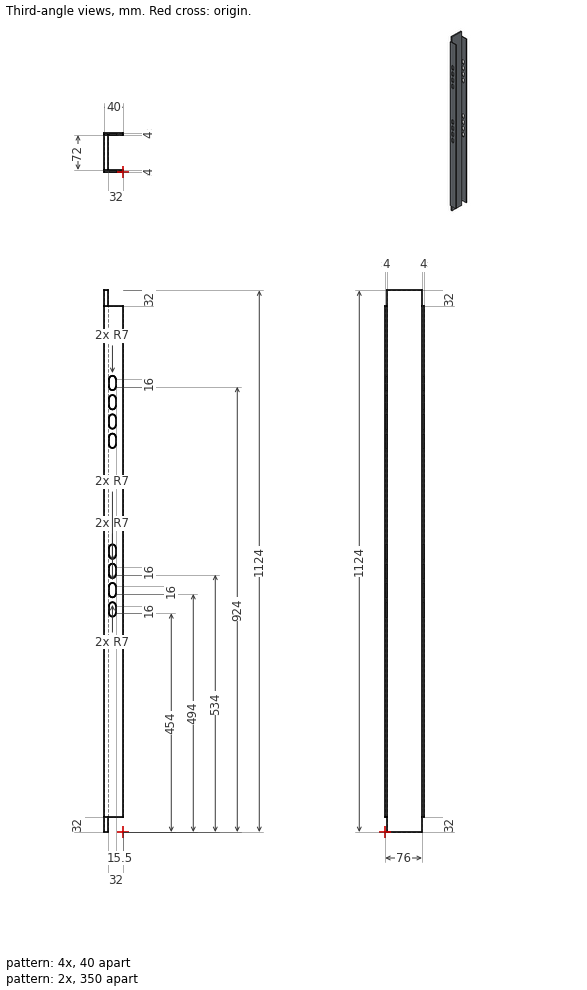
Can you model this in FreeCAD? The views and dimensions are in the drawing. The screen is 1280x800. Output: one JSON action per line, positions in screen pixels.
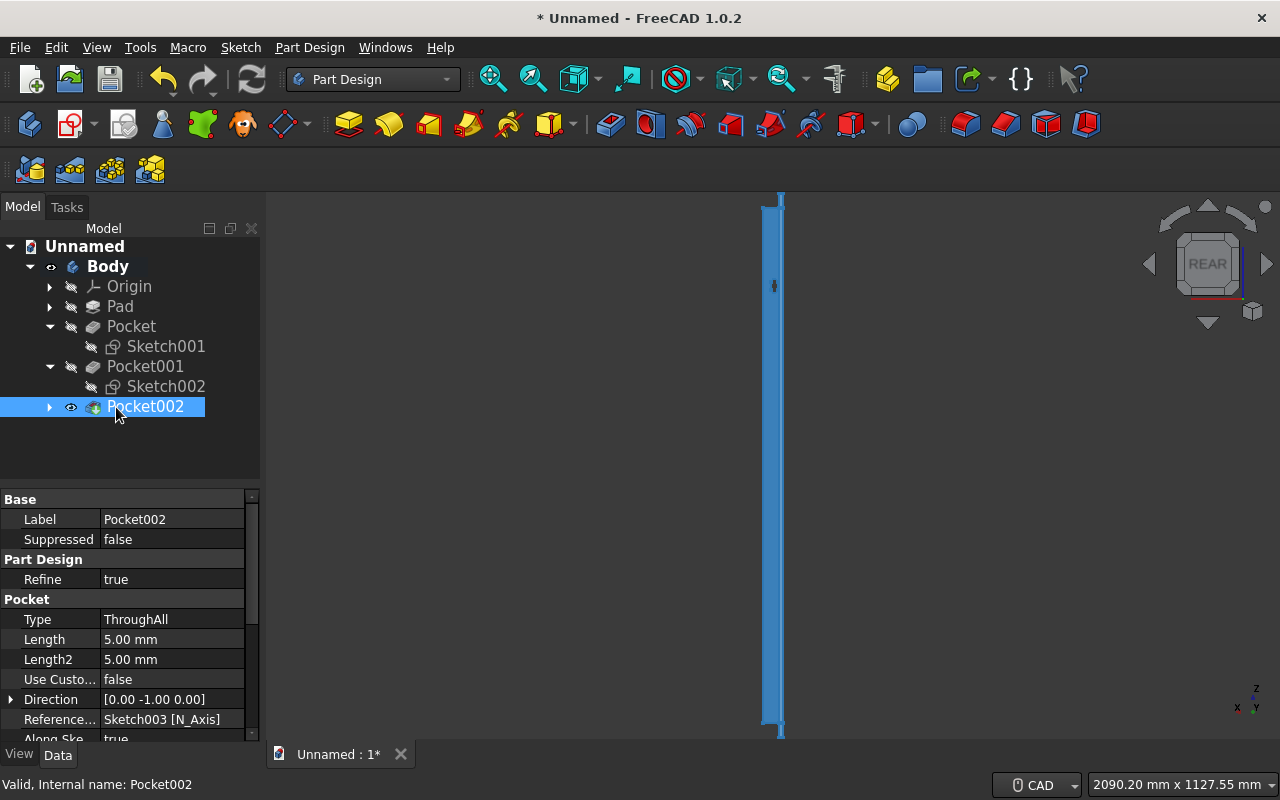
{"action": "left_click", "coordinate": [70, 170]}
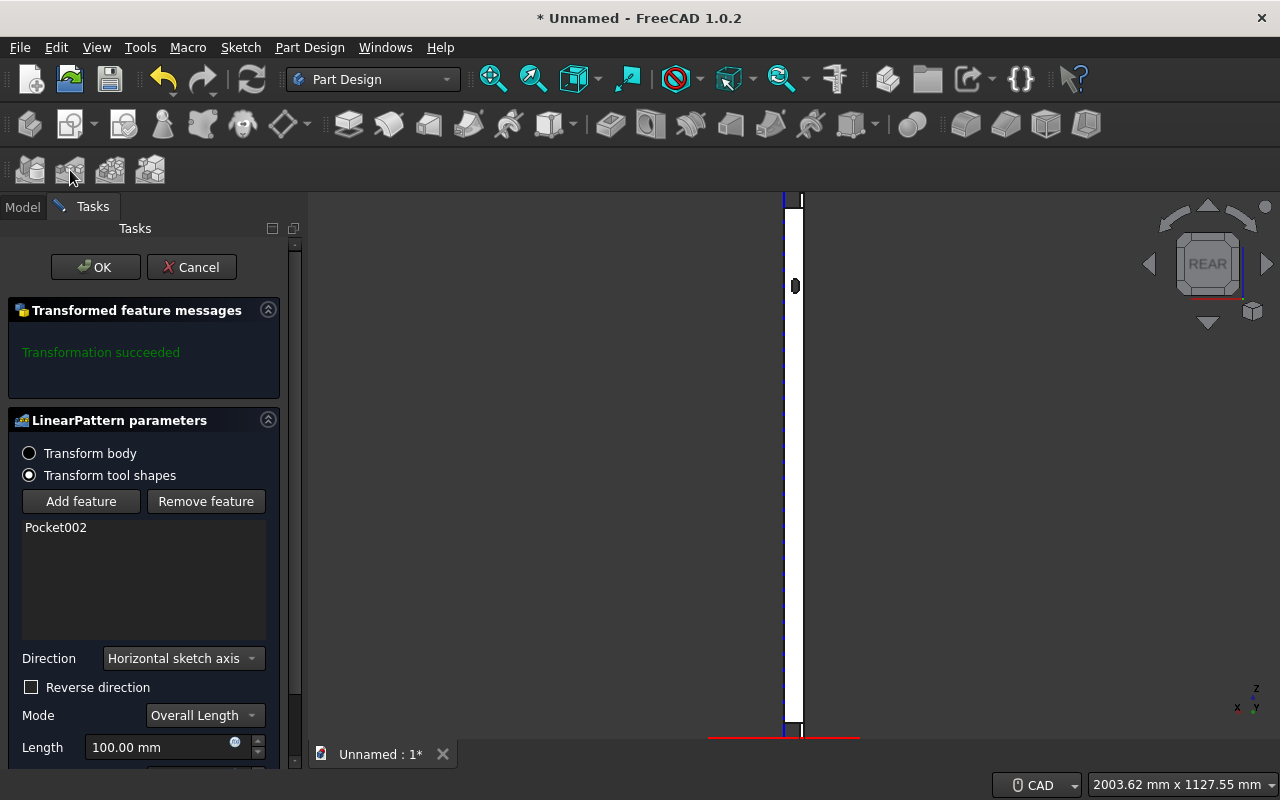
{"action": "left_click", "coordinate": [184, 658]}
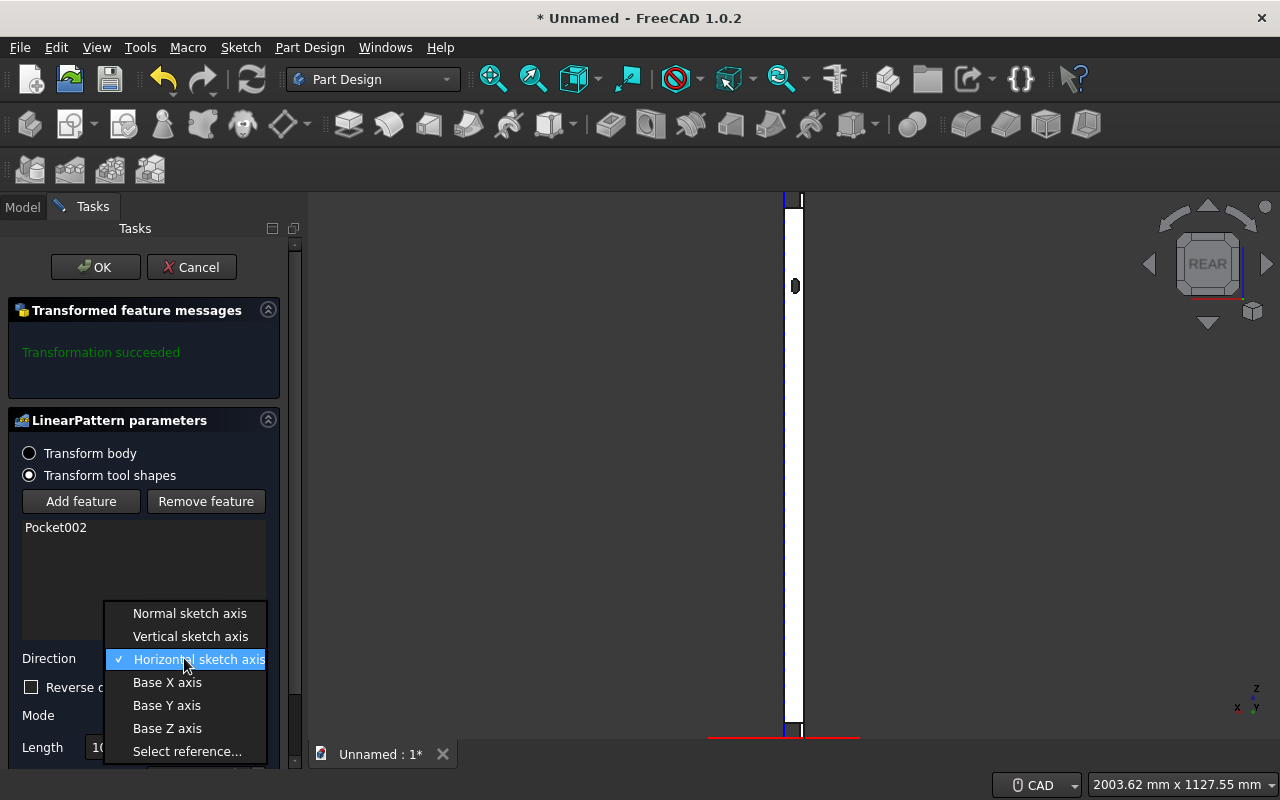
{"action": "left_click", "coordinate": [184, 728]}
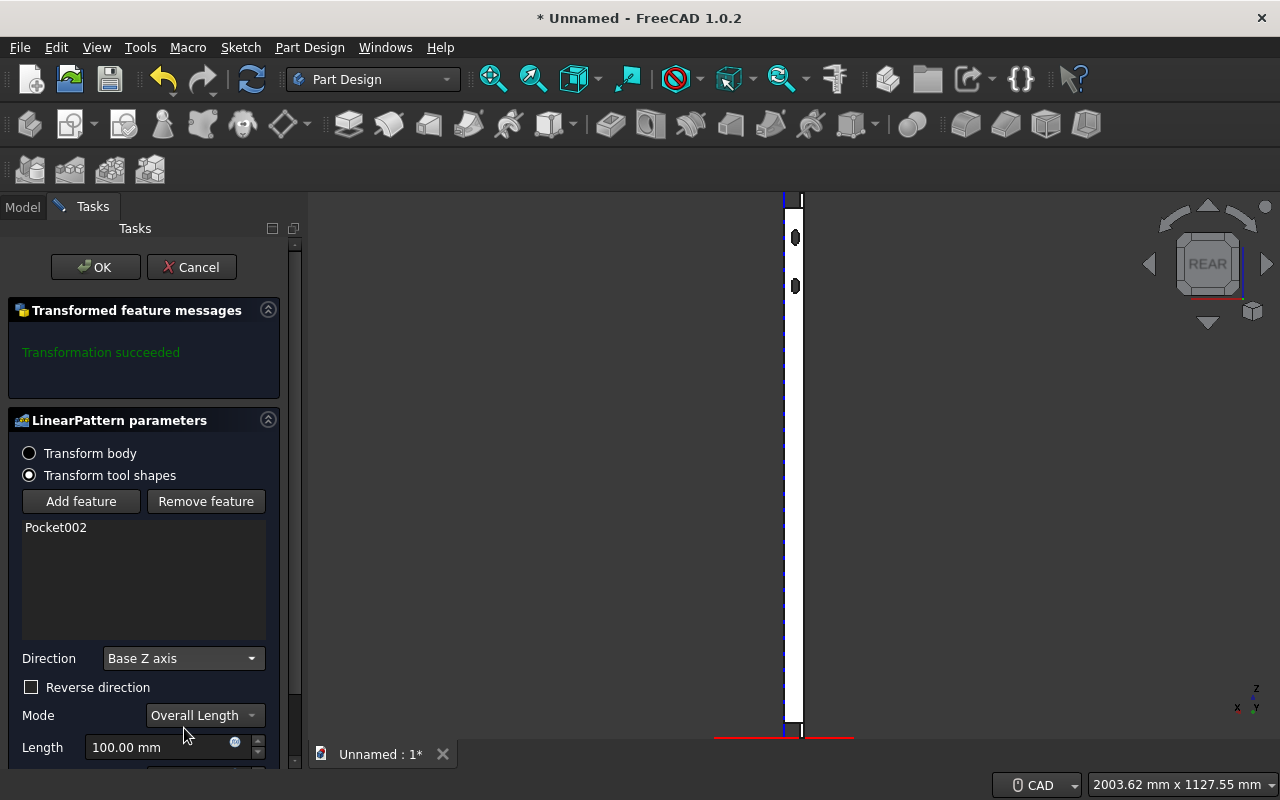
{"action": "left_click", "coordinate": [206, 716]}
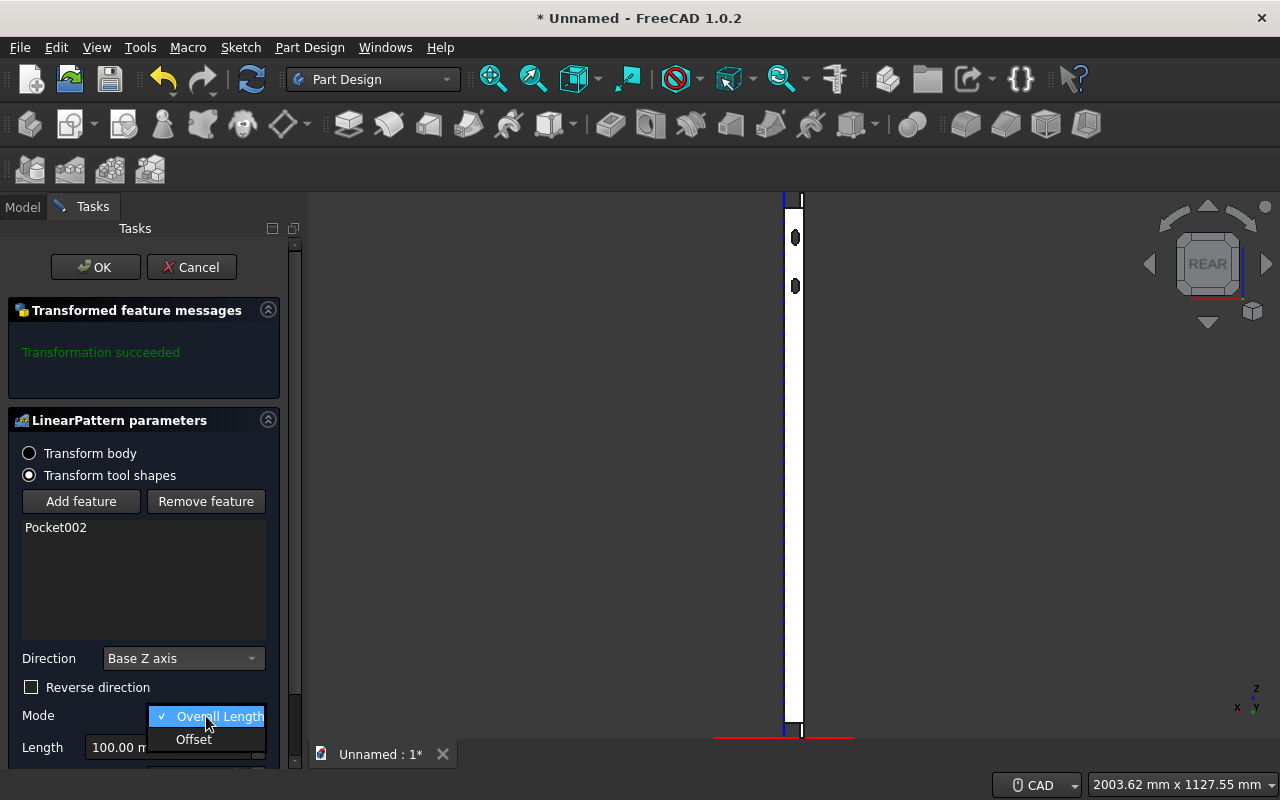
{"action": "left_click", "coordinate": [206, 740]}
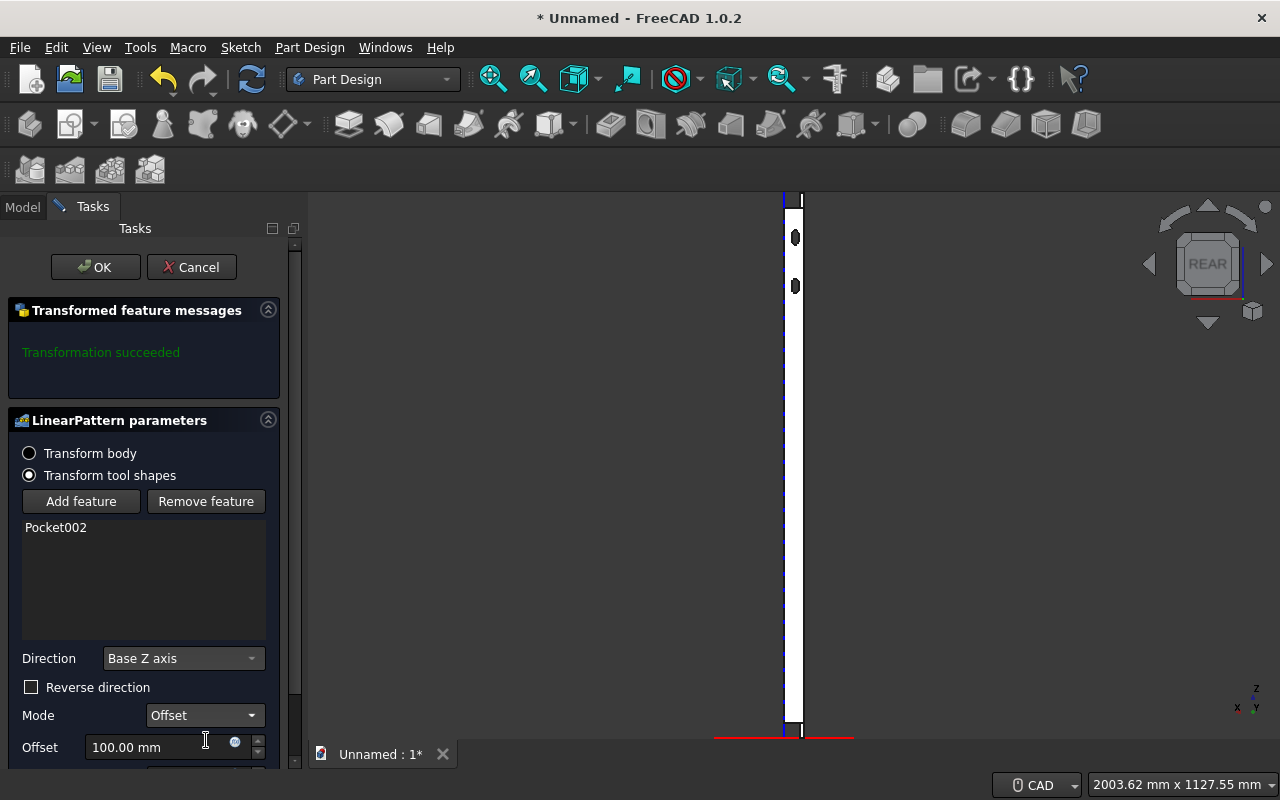
{"action": "triple_click", "coordinate": [168, 747]}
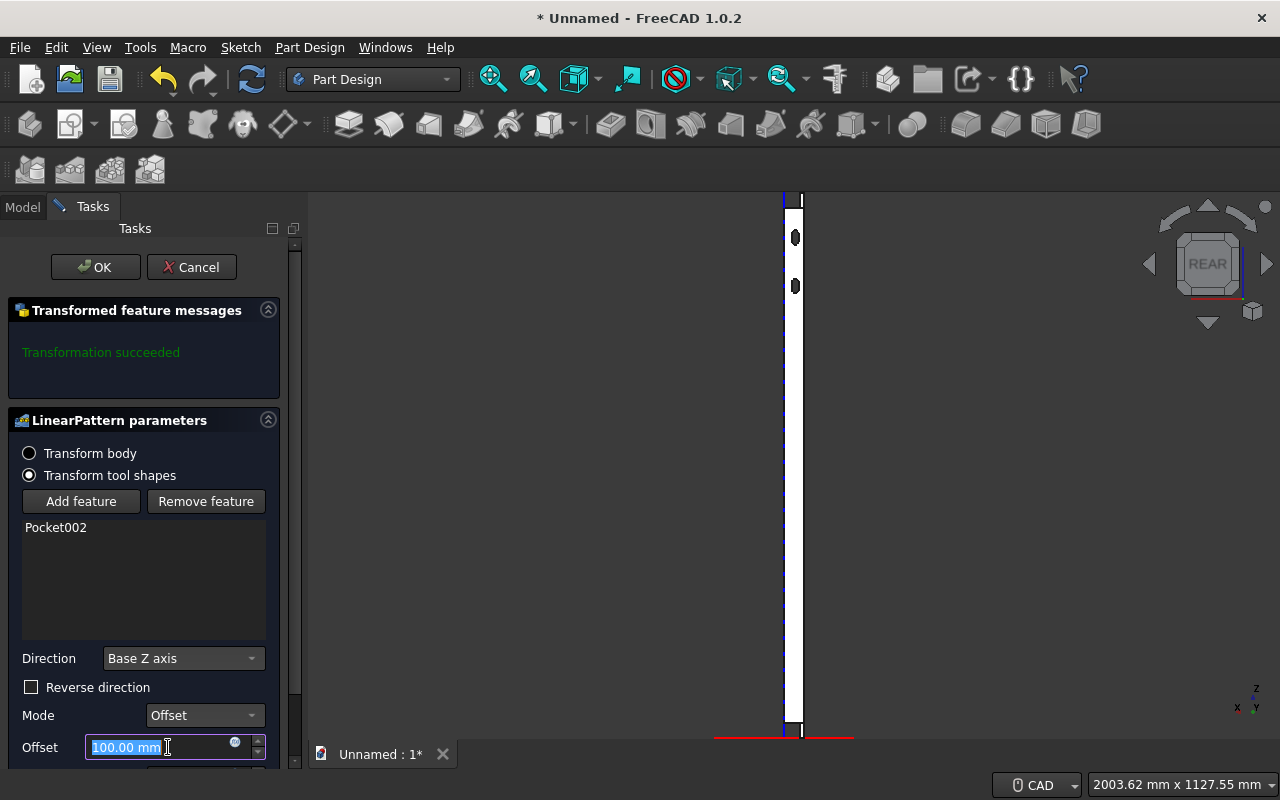
{"action": "type", "text": "40"}
{"action": "key", "text": "Tab"}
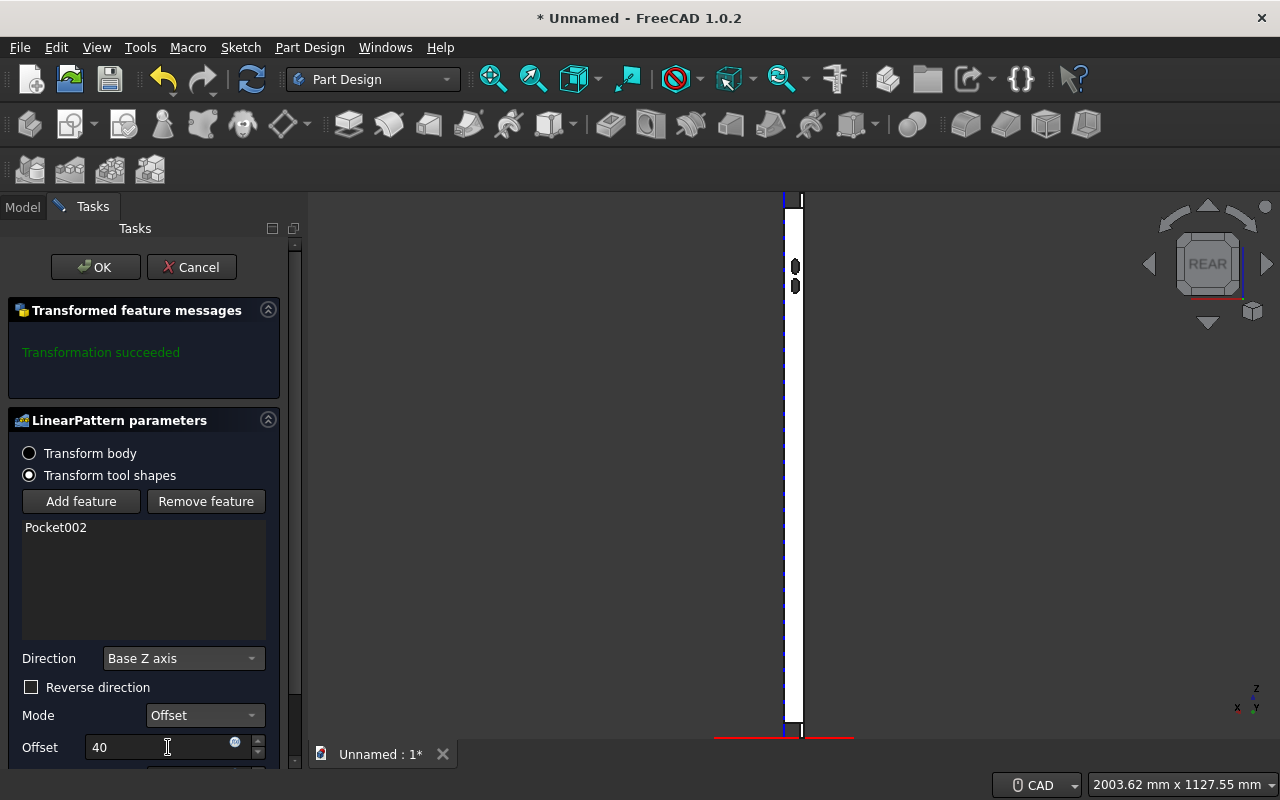
{"action": "scroll", "coordinate": [295, 503], "scroll_direction": "down", "scroll_amount": 2}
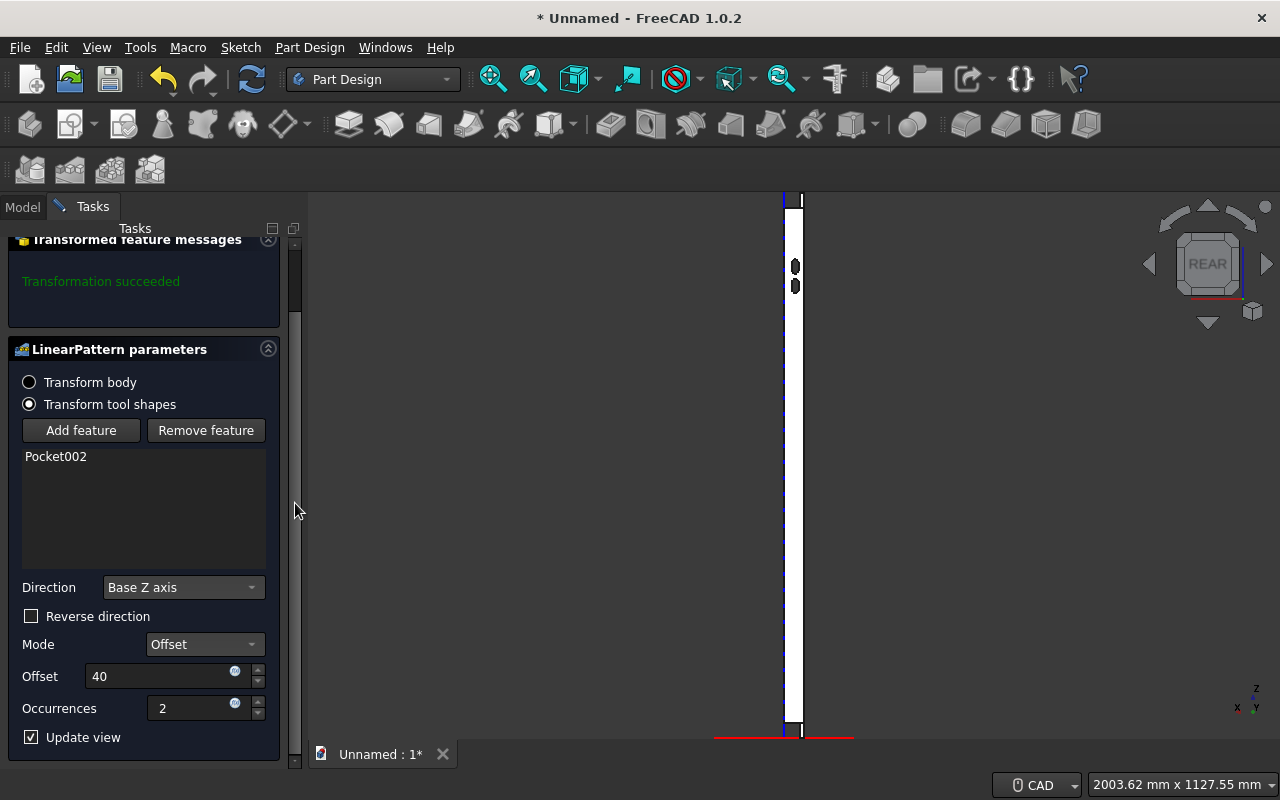
{"action": "triple_click", "coordinate": [198, 708]}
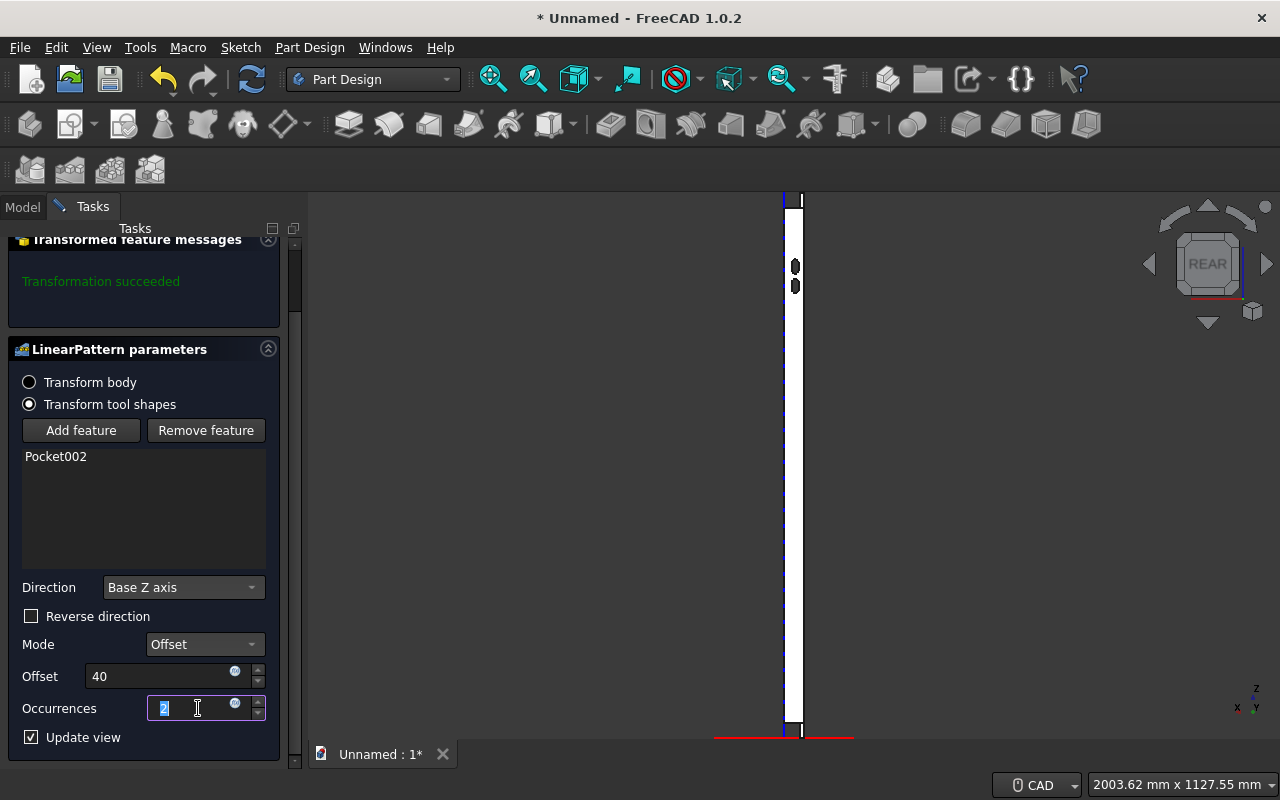
{"action": "type", "text": "4"}
{"action": "key", "text": "Tab"}